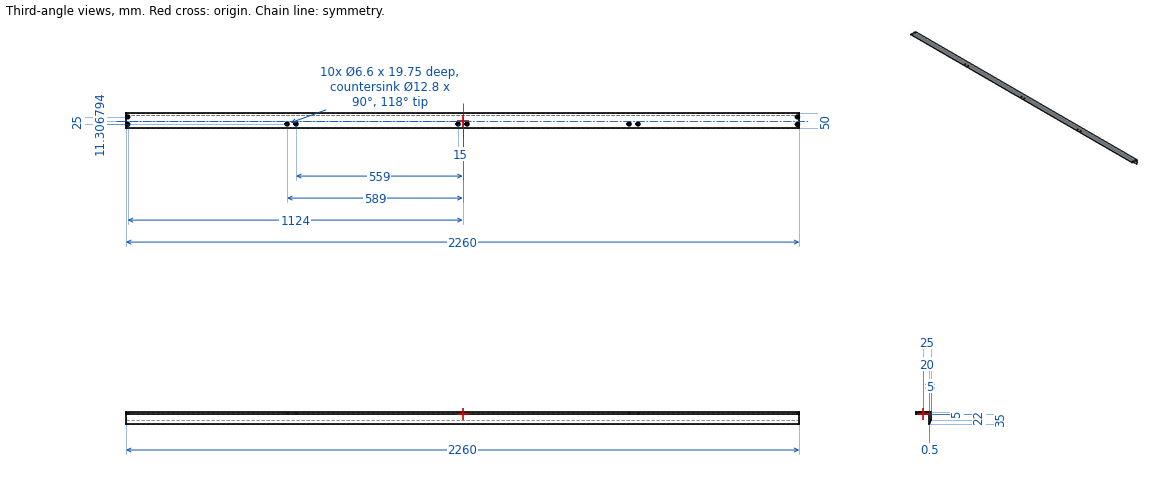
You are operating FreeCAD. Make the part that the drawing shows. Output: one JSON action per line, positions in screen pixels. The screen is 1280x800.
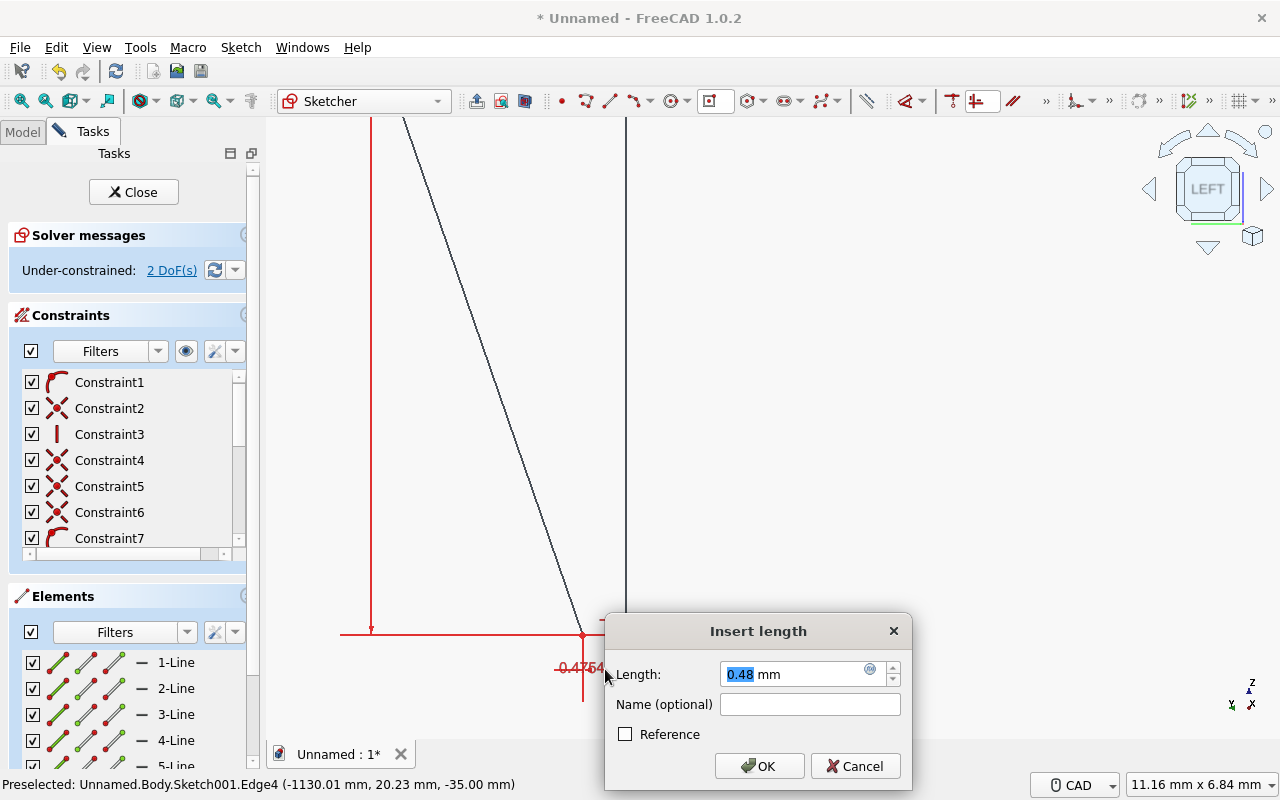
{"action": "type", "text": "0.5"}
{"action": "key", "text": "Return"}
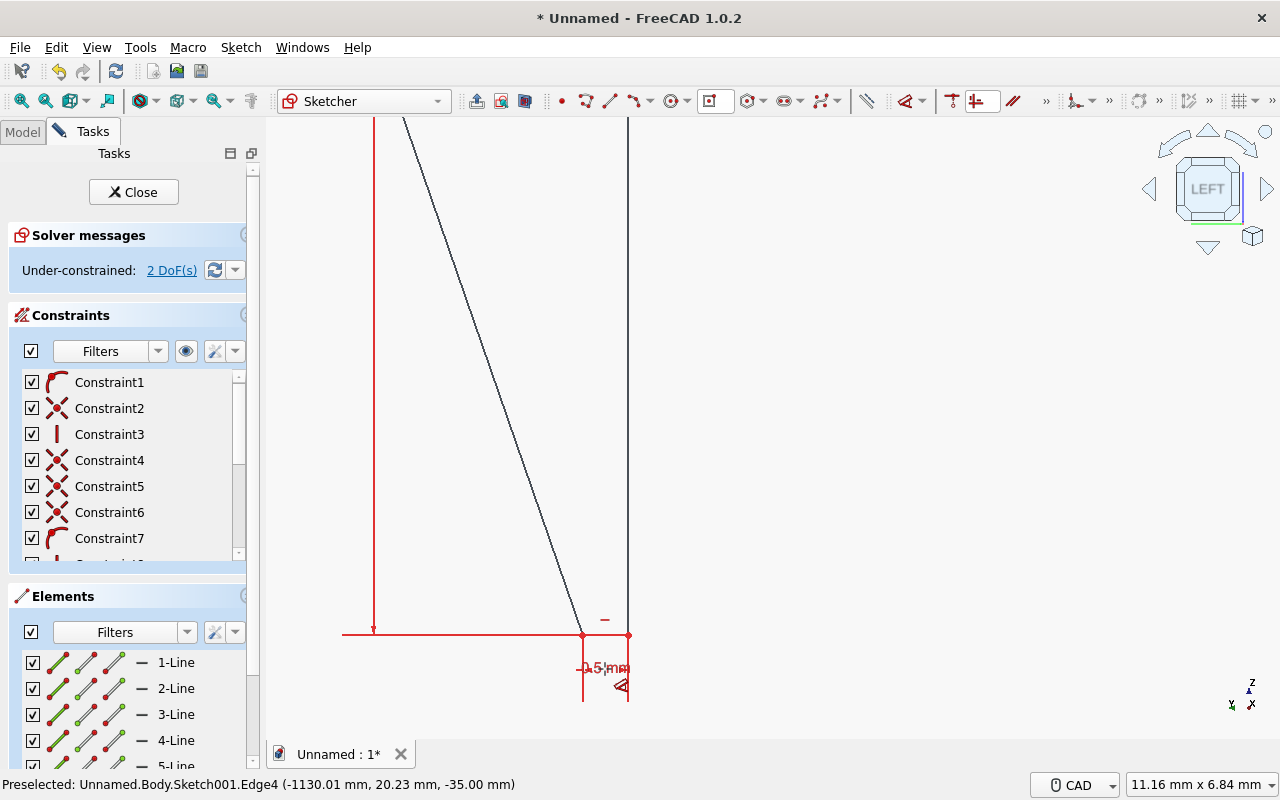
{"action": "scroll", "coordinate": [610, 644], "scroll_direction": "down", "scroll_amount": 10}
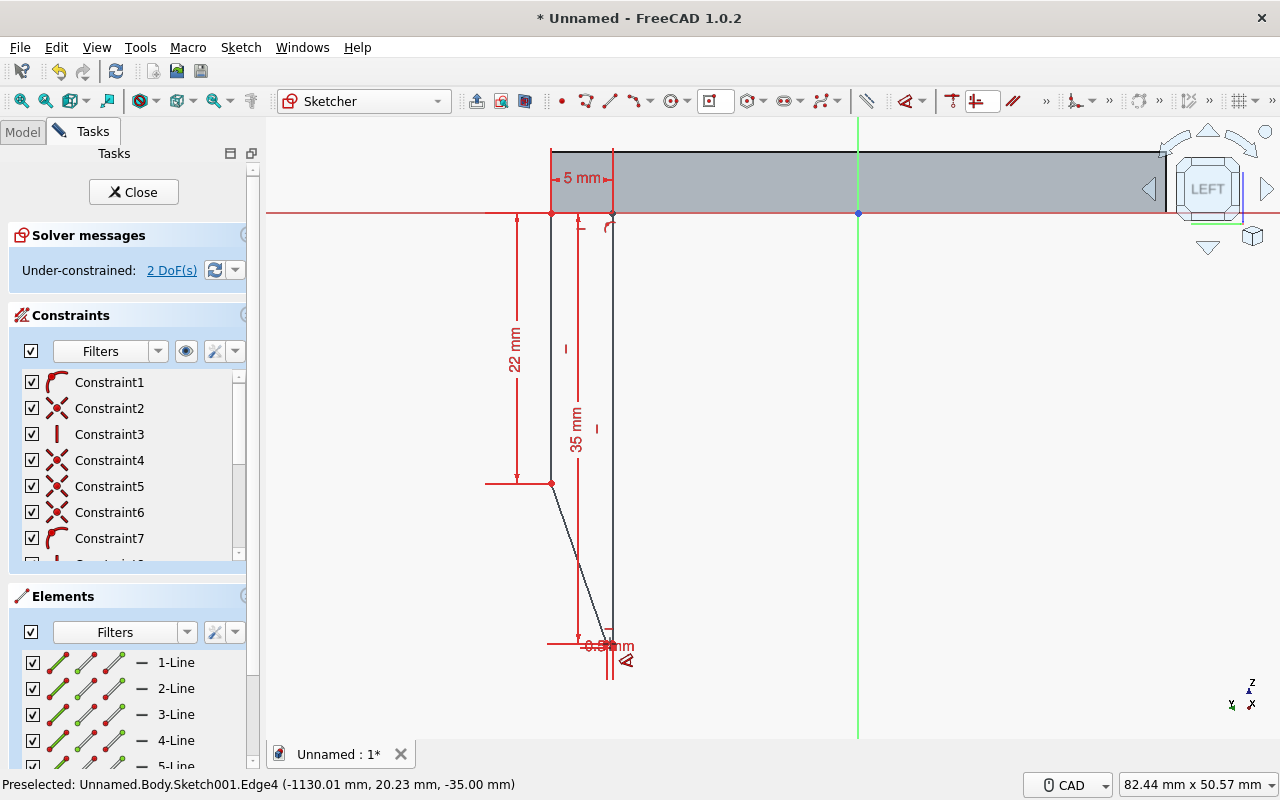
{"action": "left_click", "coordinate": [613, 213]}
{"action": "left_click", "coordinate": [736, 179]}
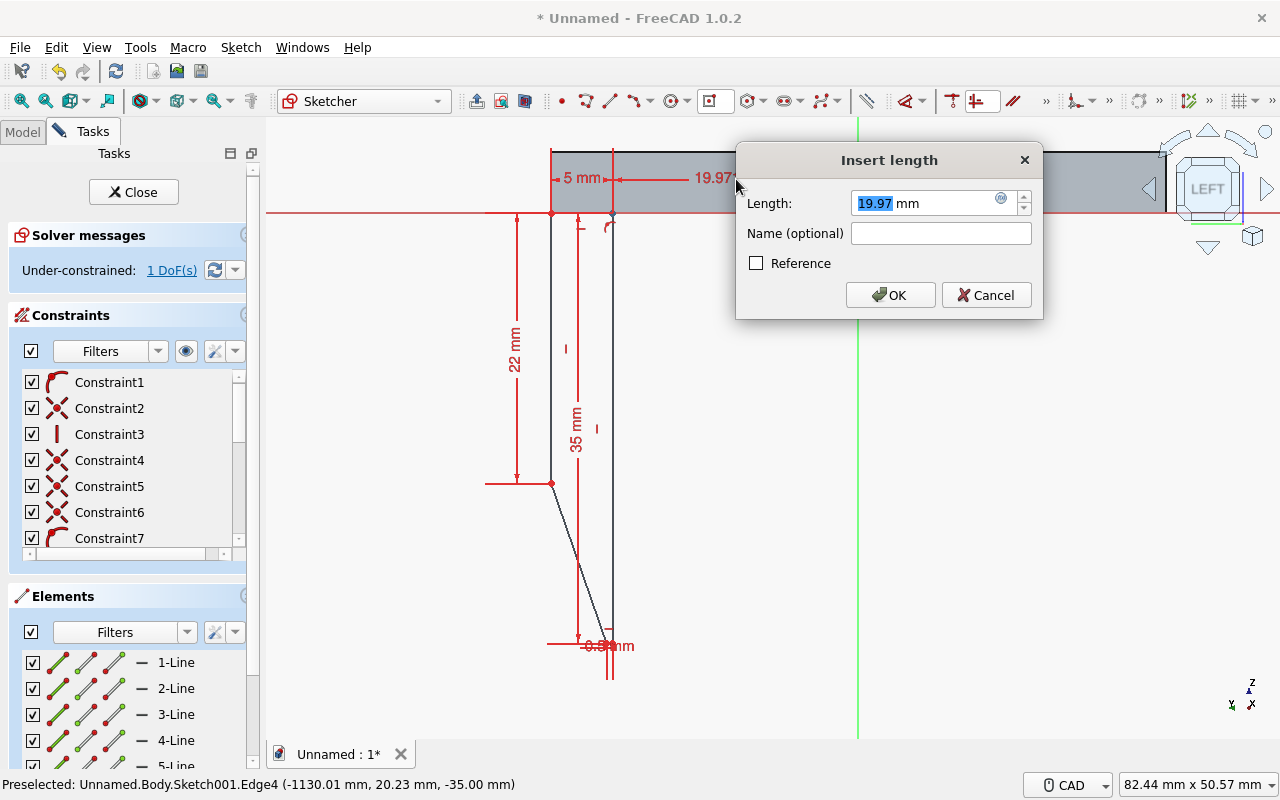
{"action": "type", "text": "20"}
{"action": "key", "text": "Return"}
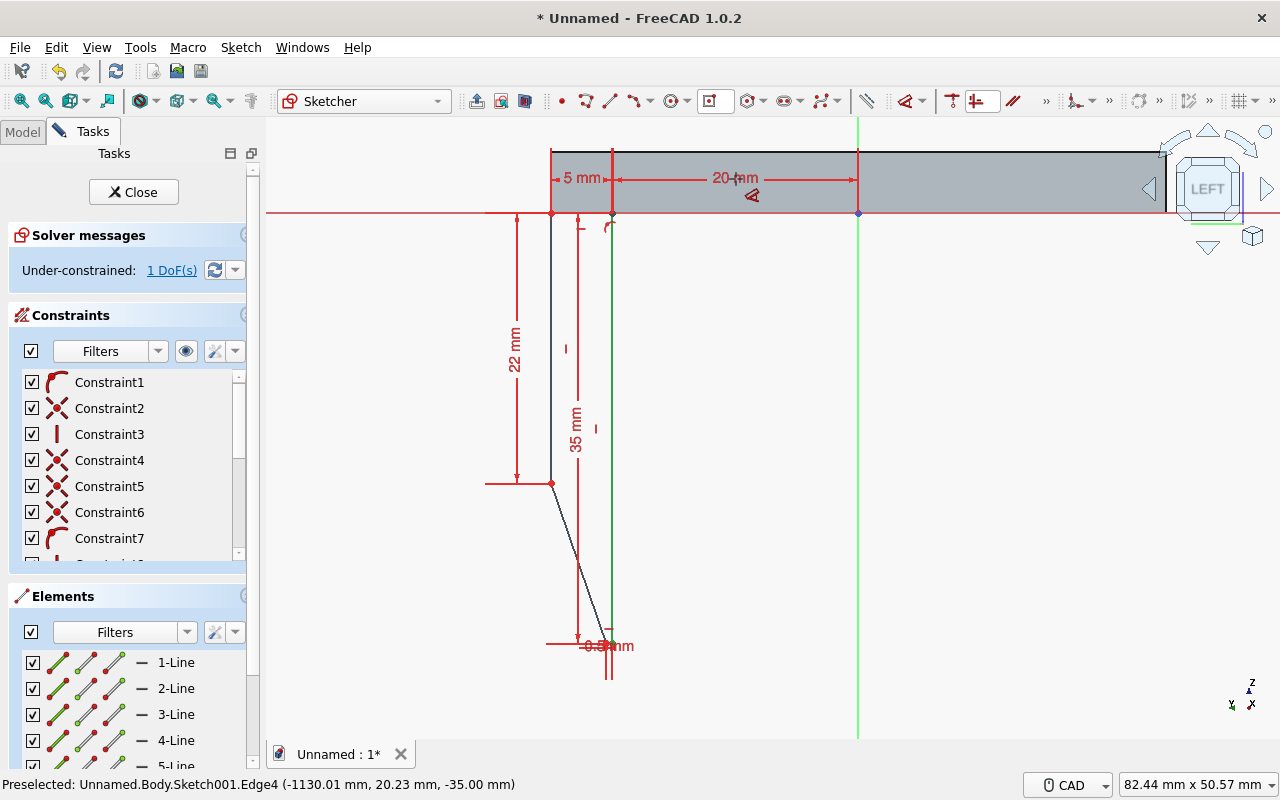
{"action": "left_click", "coordinate": [551, 213]}
{"action": "left_click", "coordinate": [812, 179]}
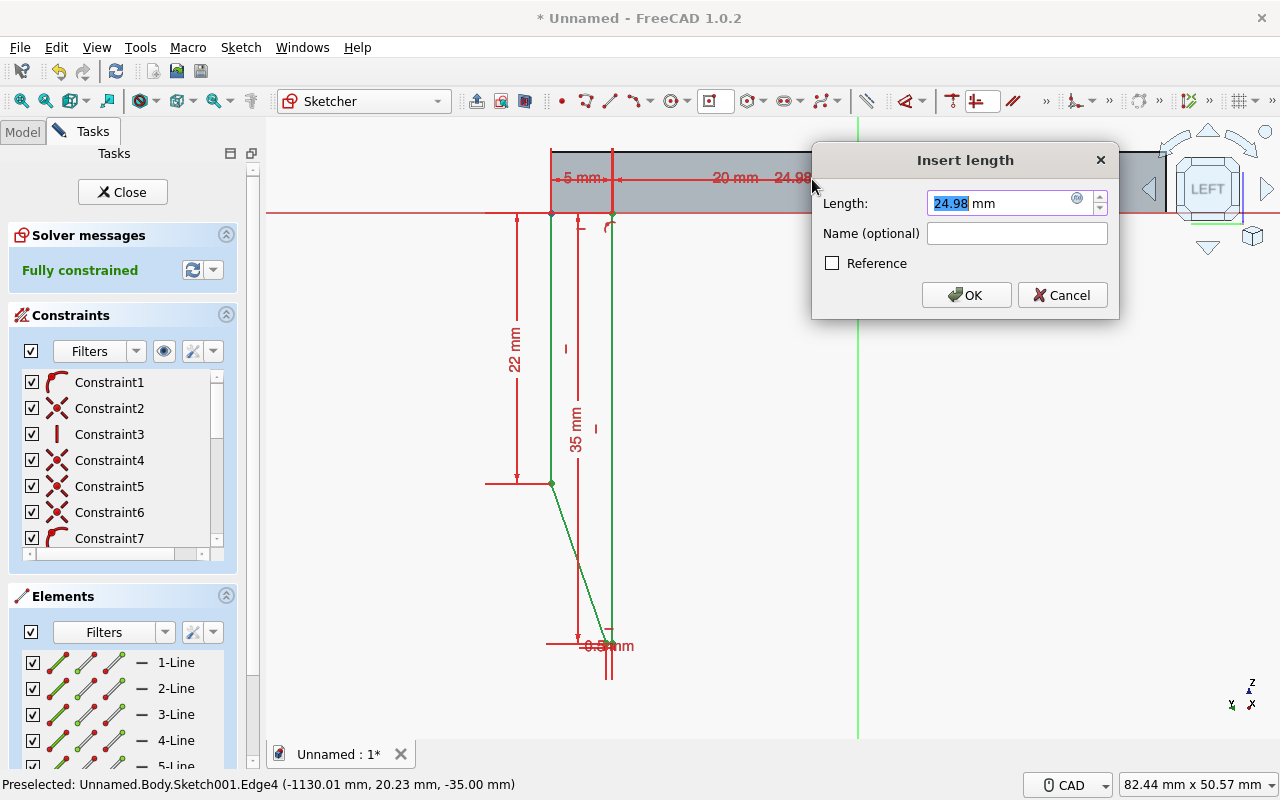
{"action": "type", "text": "25"}
{"action": "key", "text": "Return"}
{"action": "key", "text": "Escape"}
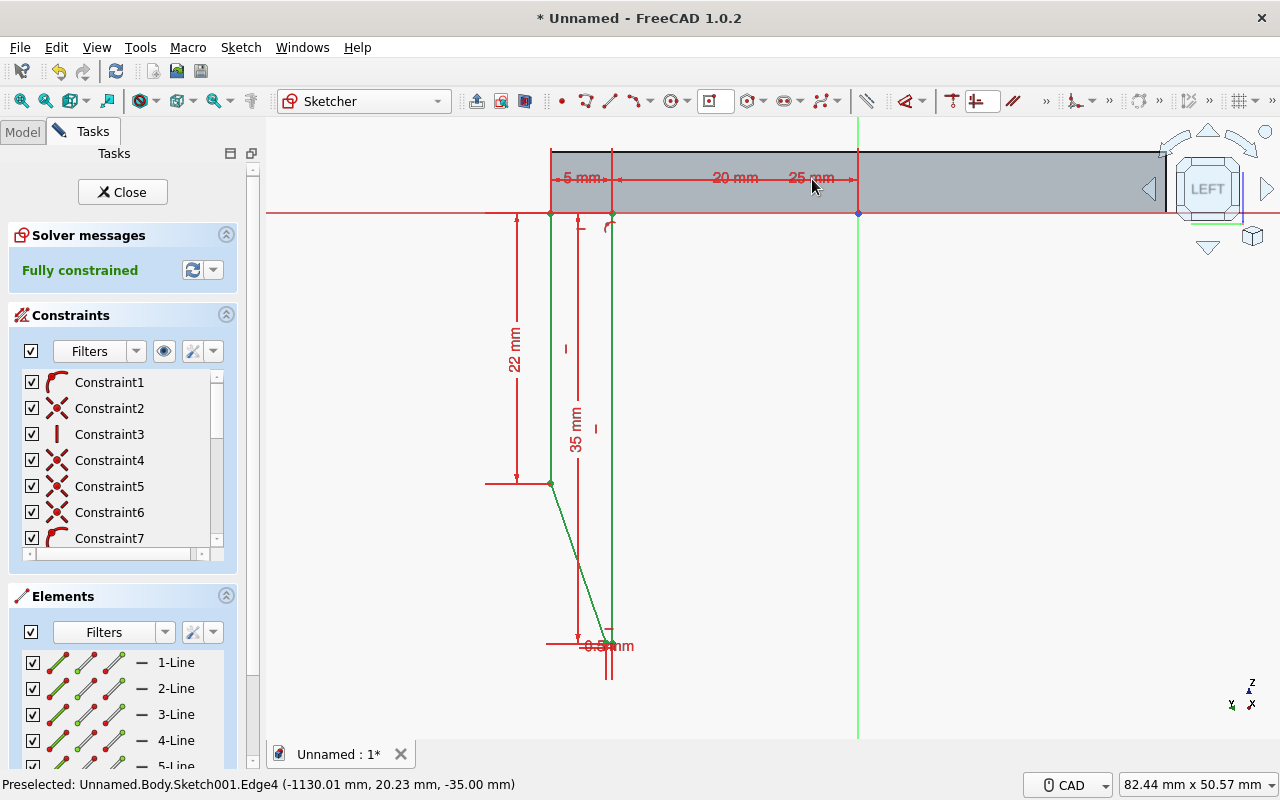
{"action": "left_click", "coordinate": [123, 192]}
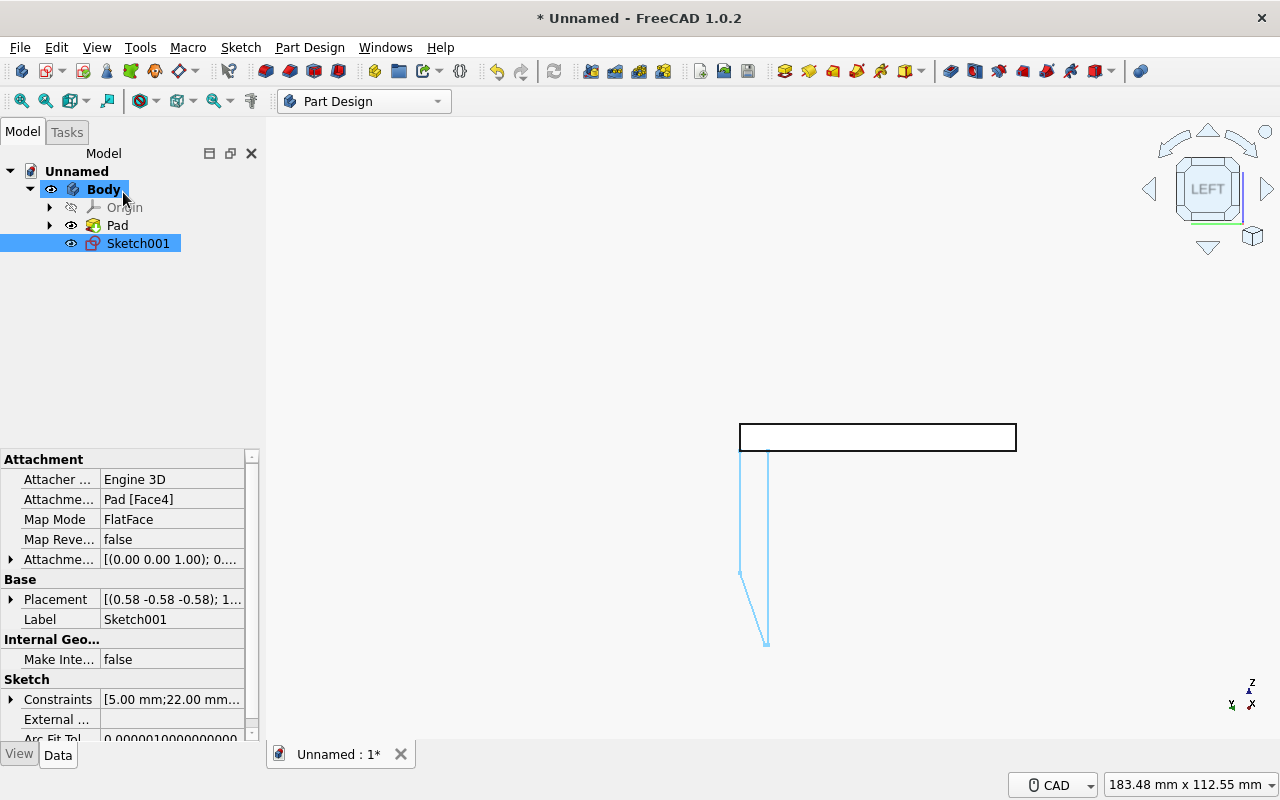
{"action": "left_click", "coordinate": [786, 72]}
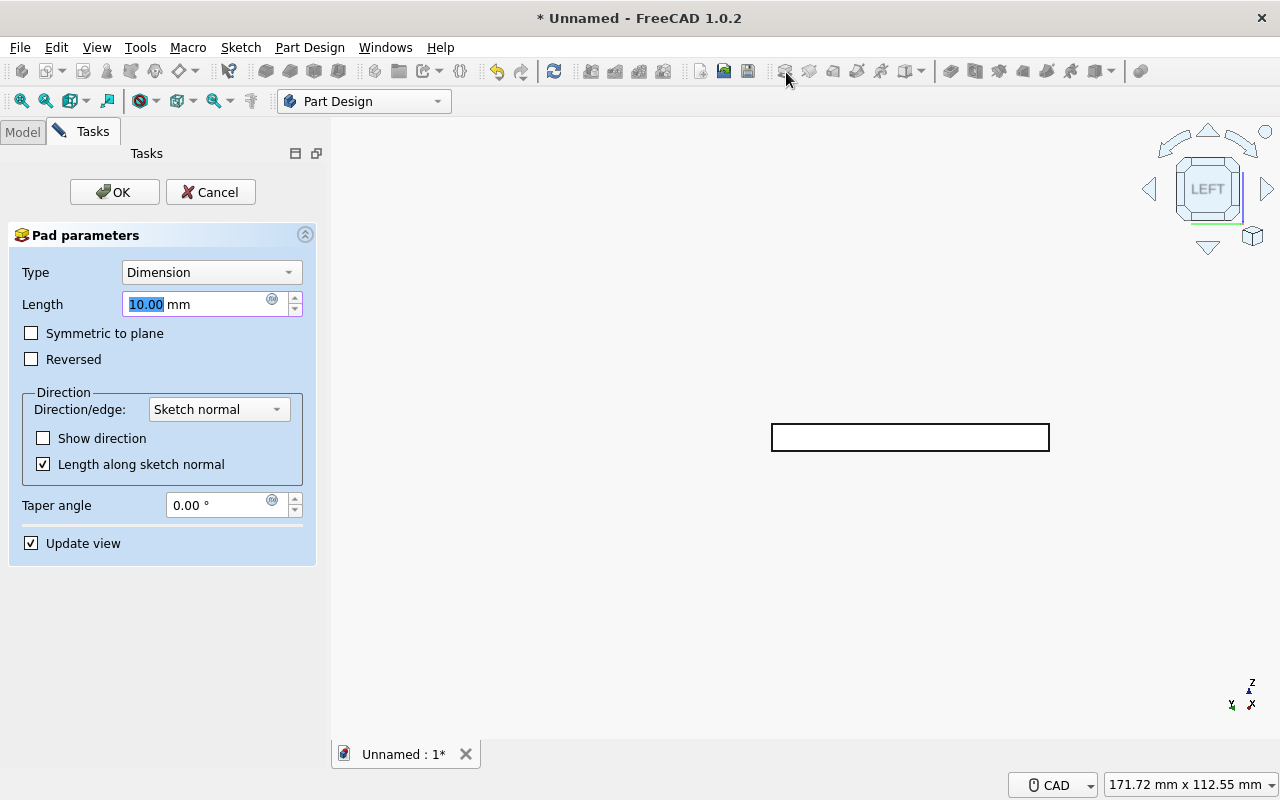
{"action": "type", "text": "2260"}
{"action": "key", "text": "Tab"}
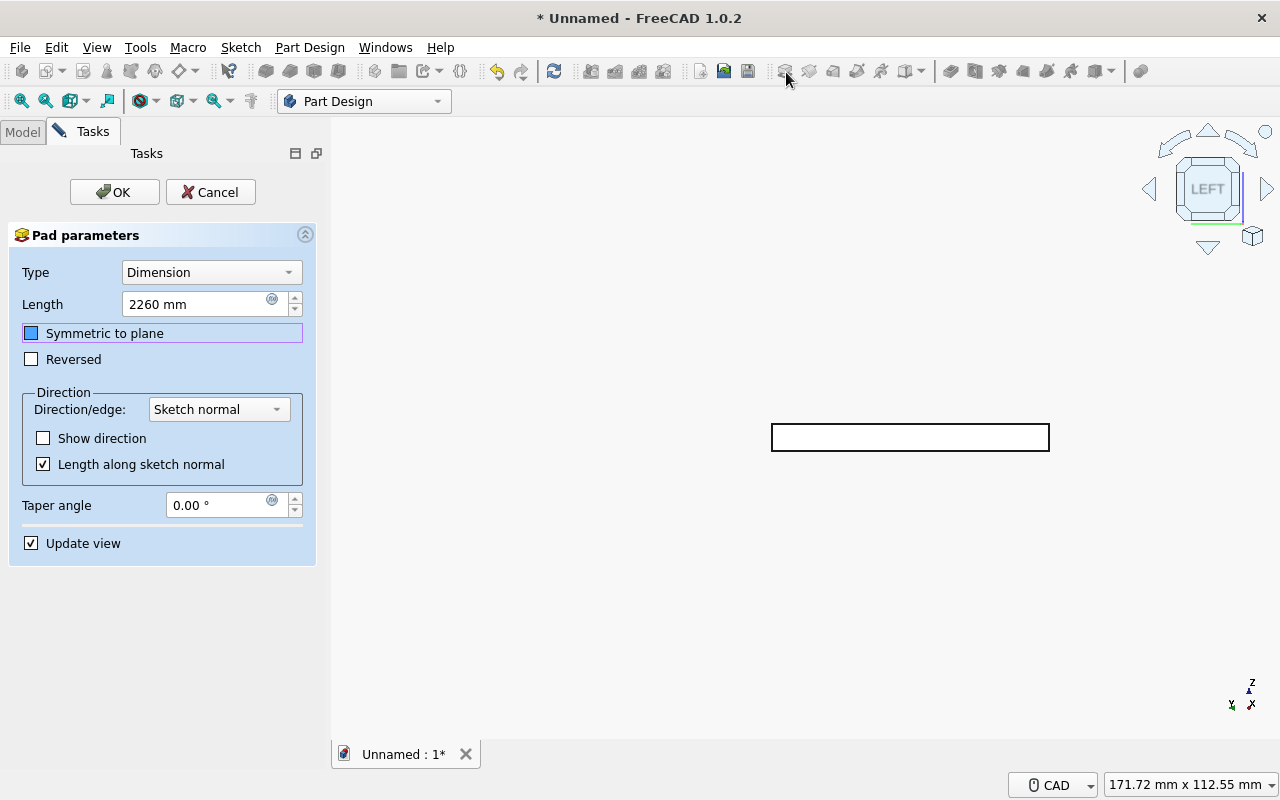
{"action": "left_click", "coordinate": [30, 359]}